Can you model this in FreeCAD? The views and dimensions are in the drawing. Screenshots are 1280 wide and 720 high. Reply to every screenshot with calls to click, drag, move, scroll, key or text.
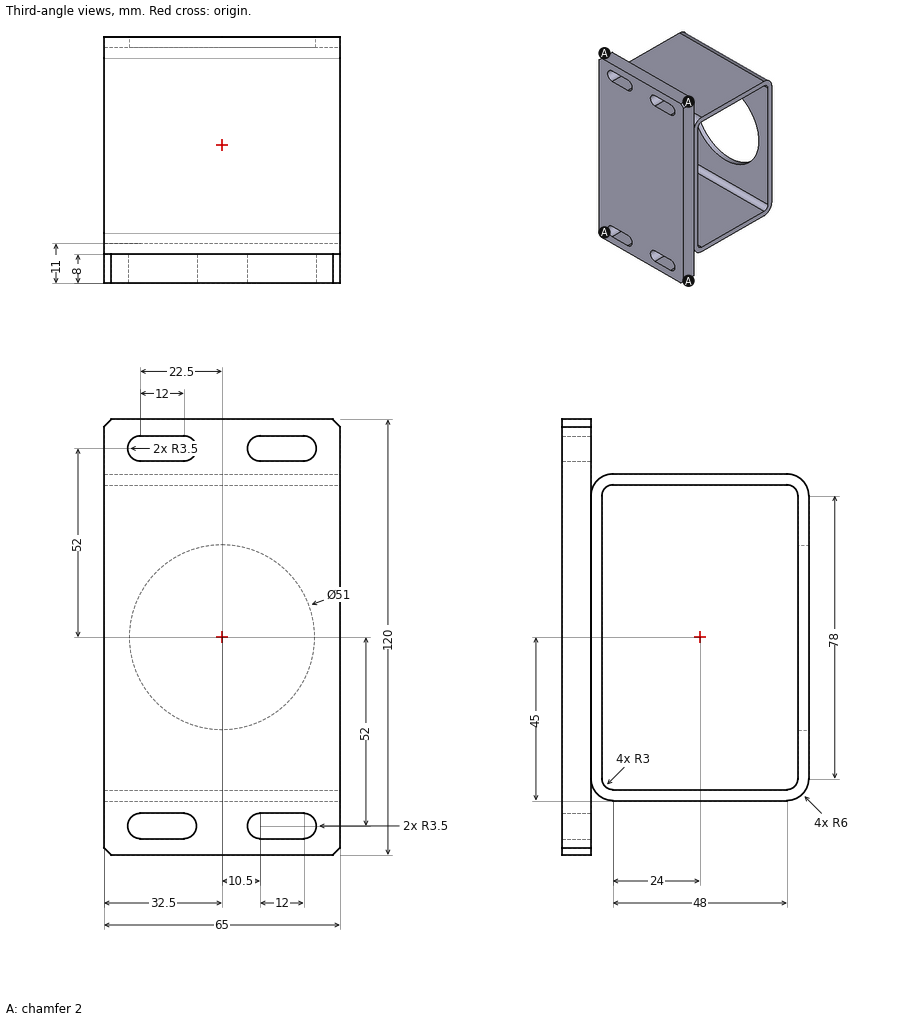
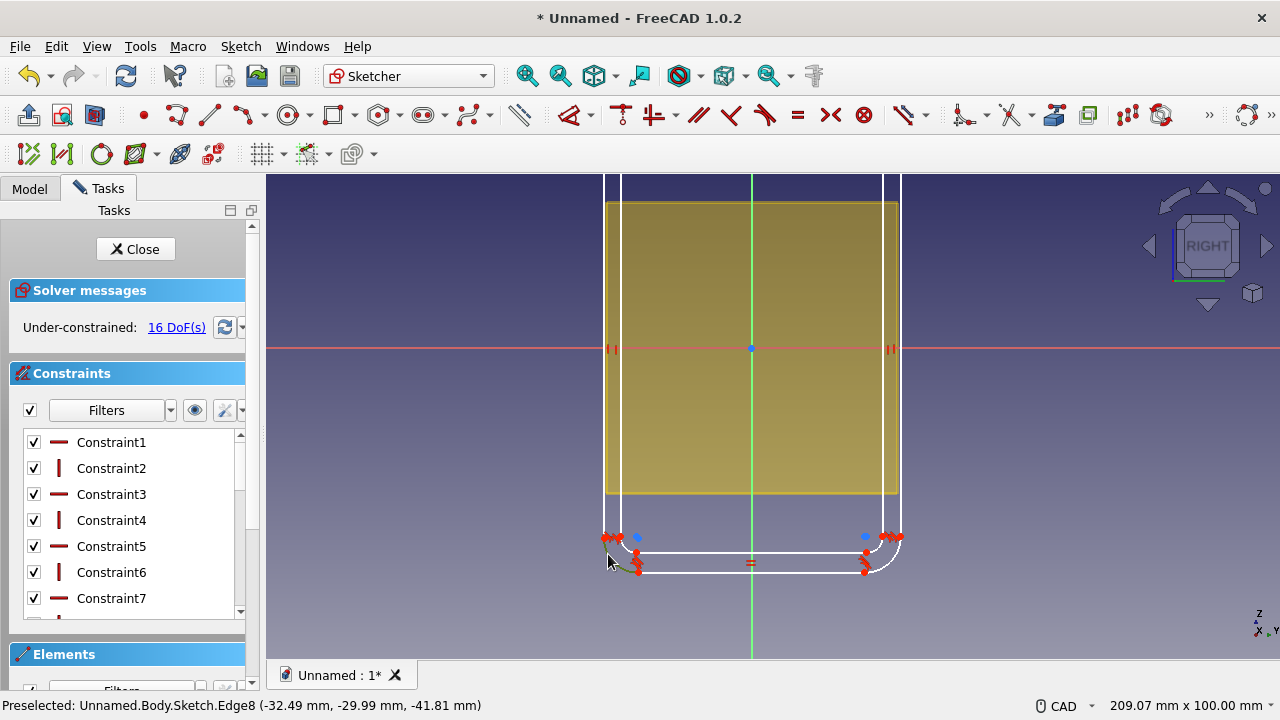
click(625, 548)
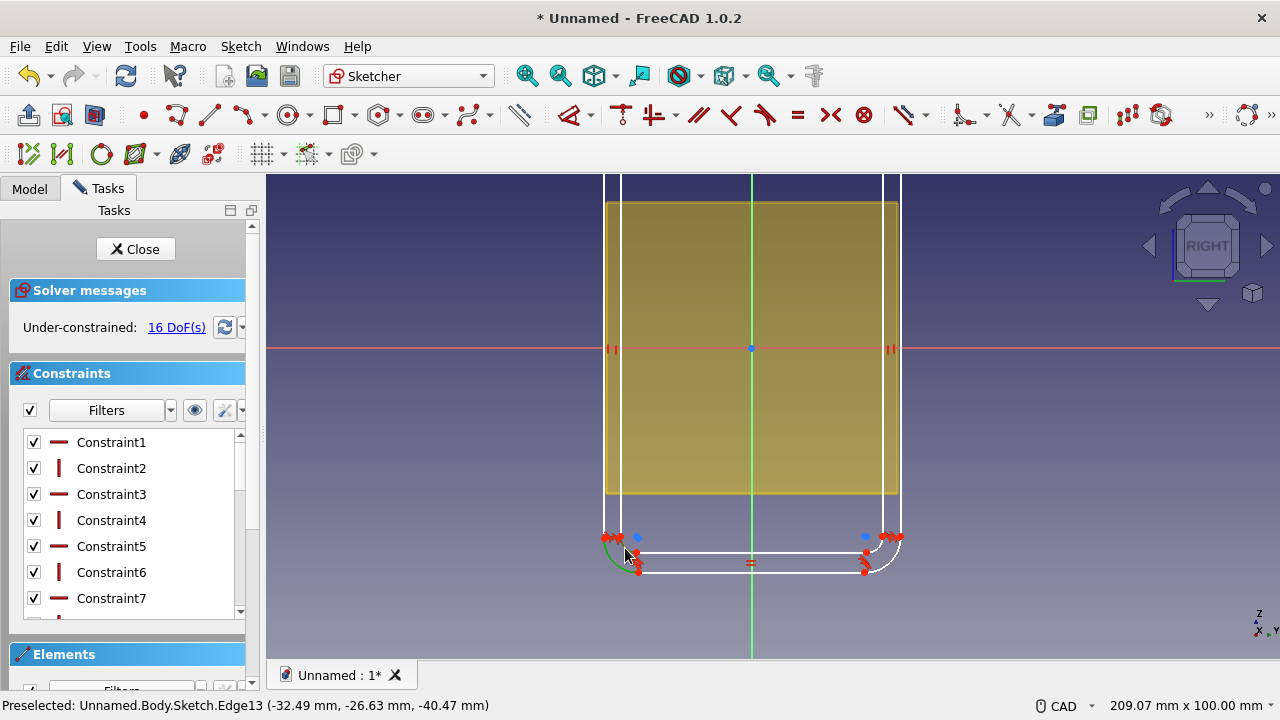
click(621, 116)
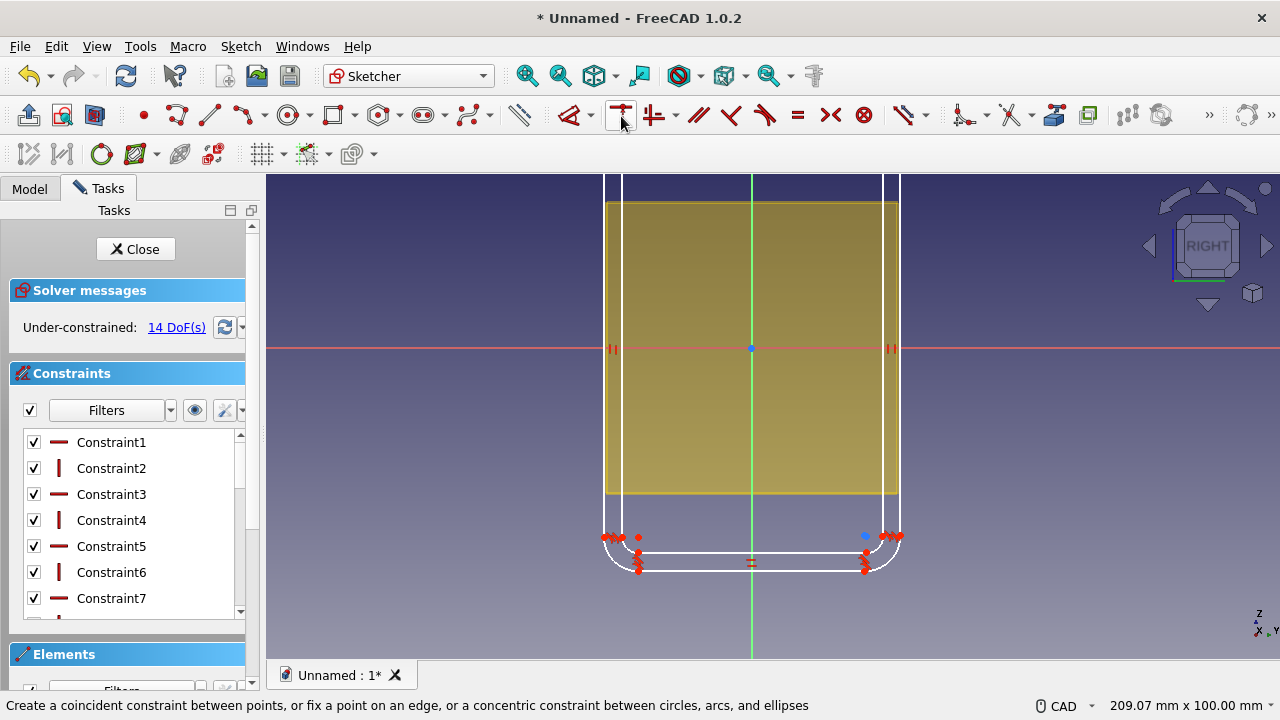
scroll(608, 555, down, 2)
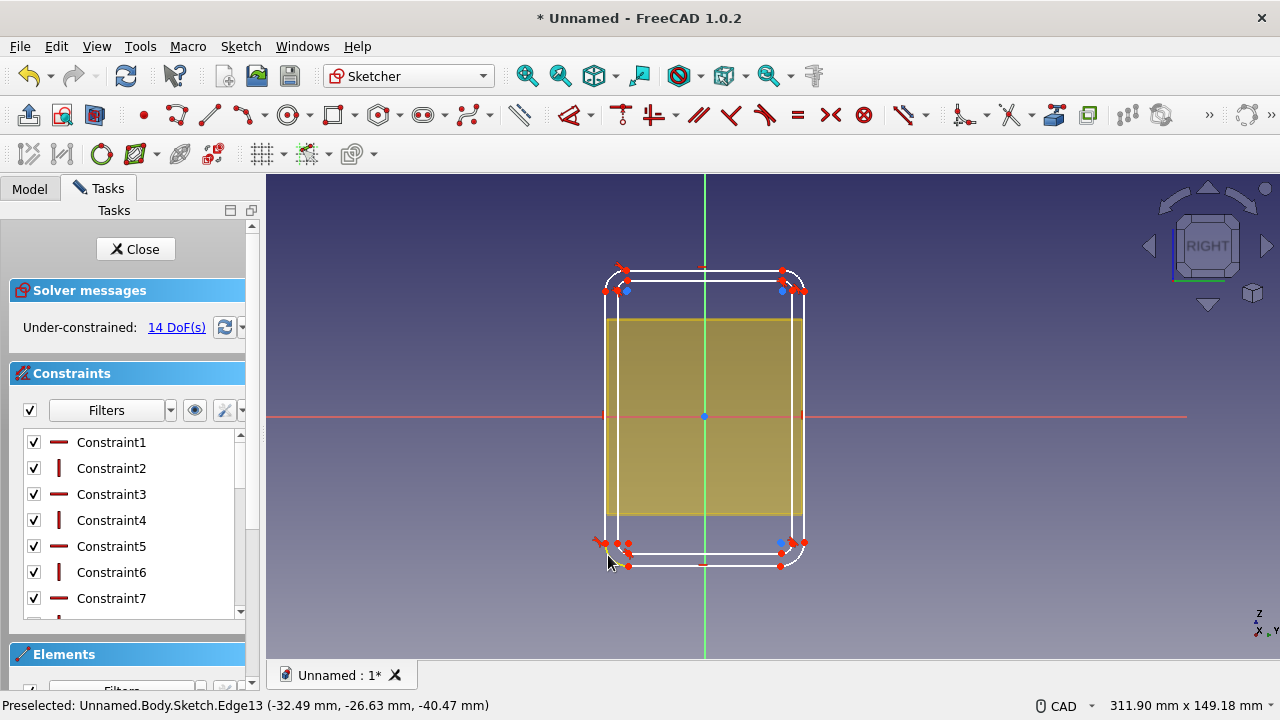
scroll(617, 273, up, 2)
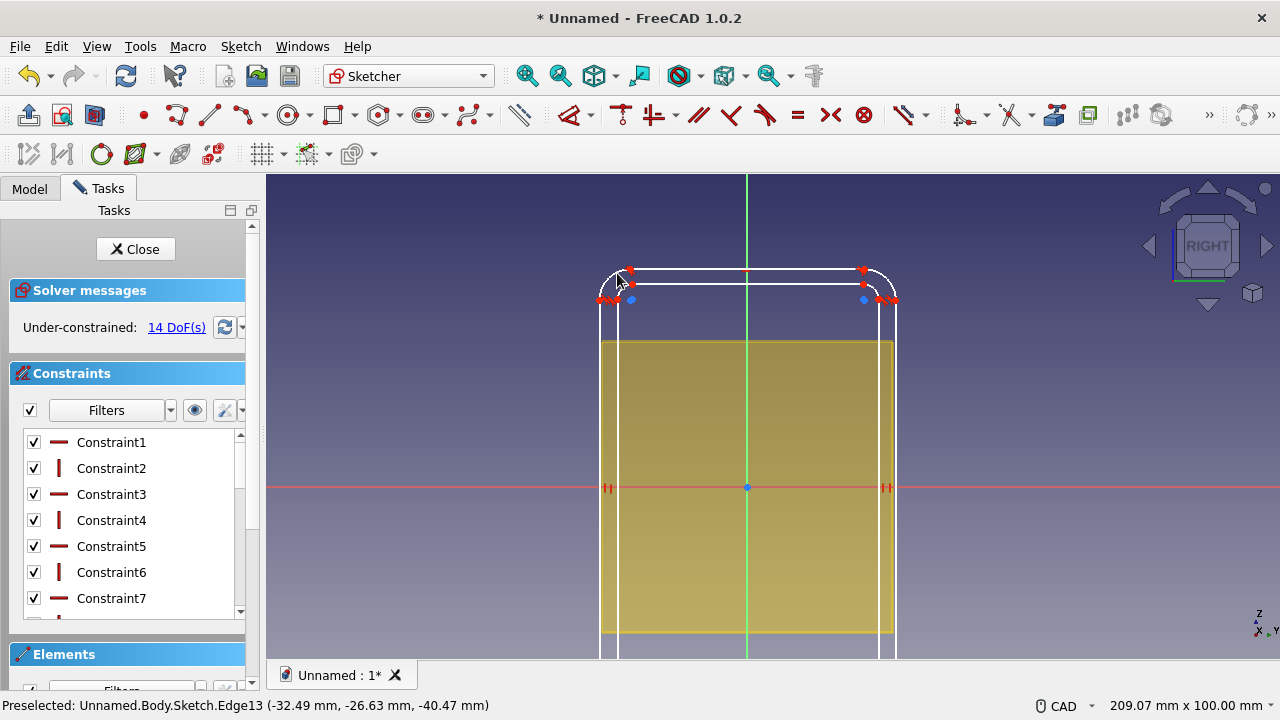
click(616, 273)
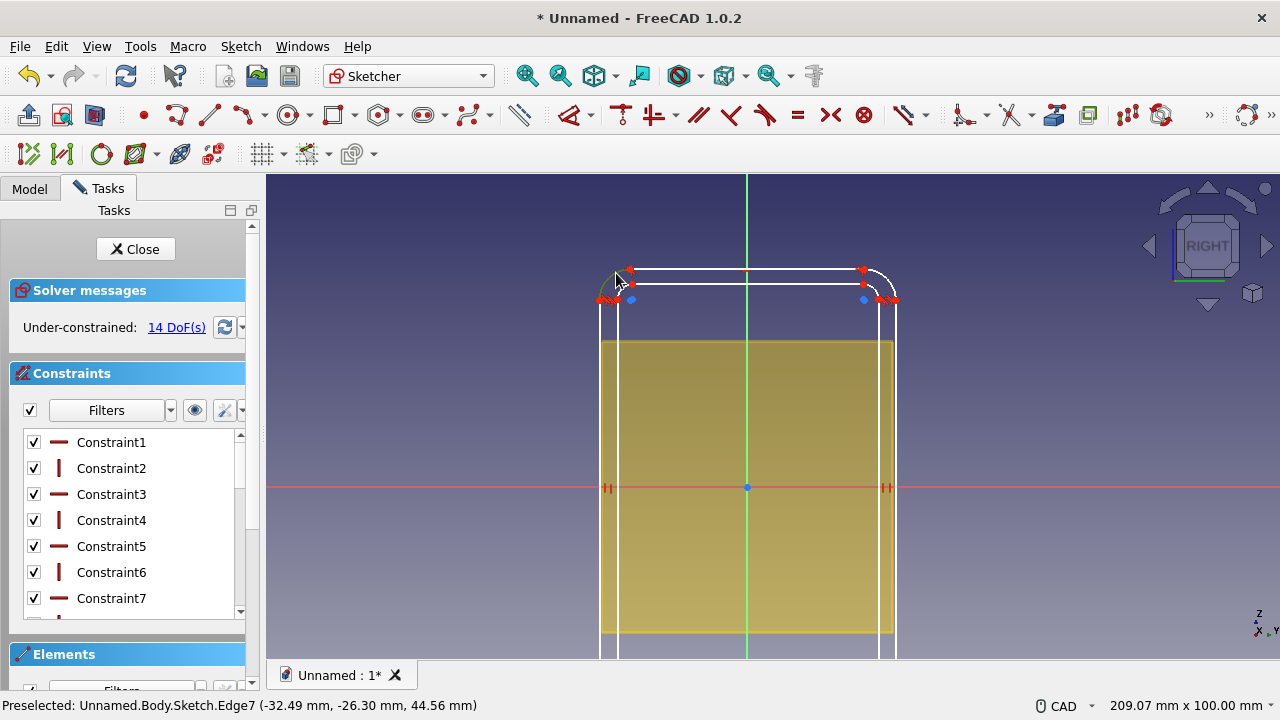
scroll(622, 289, up, 2)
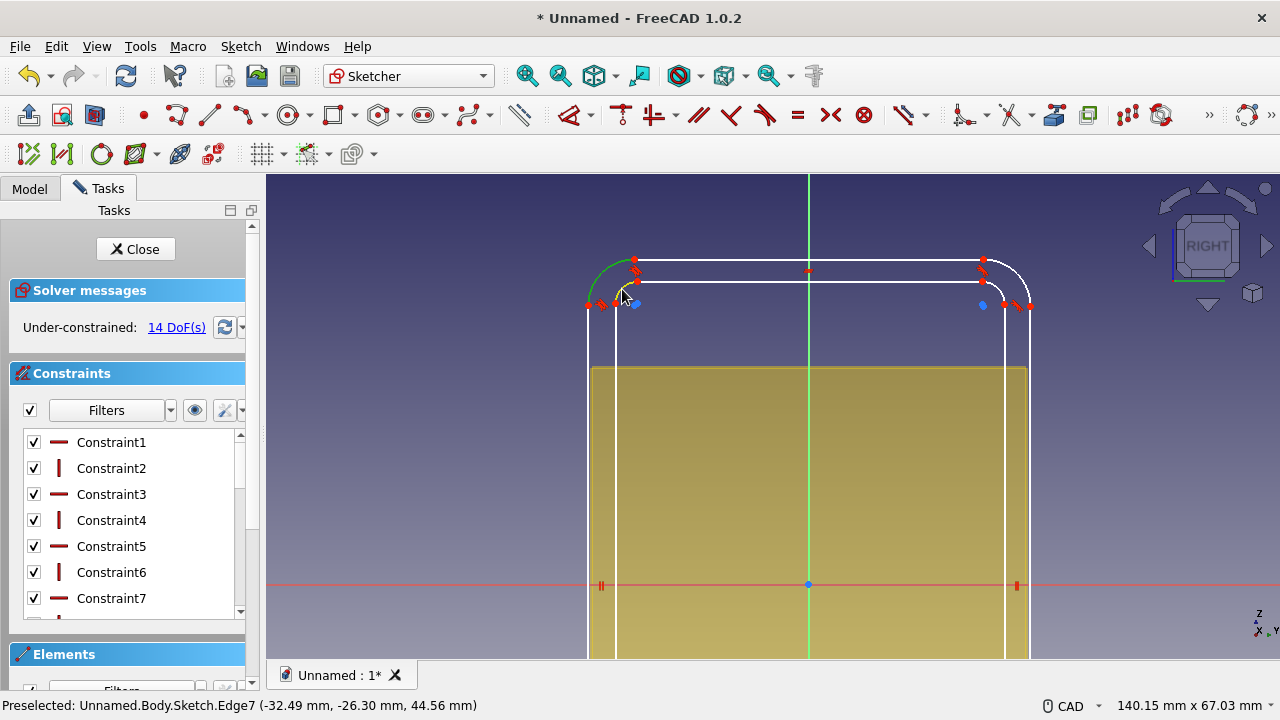
click(622, 288)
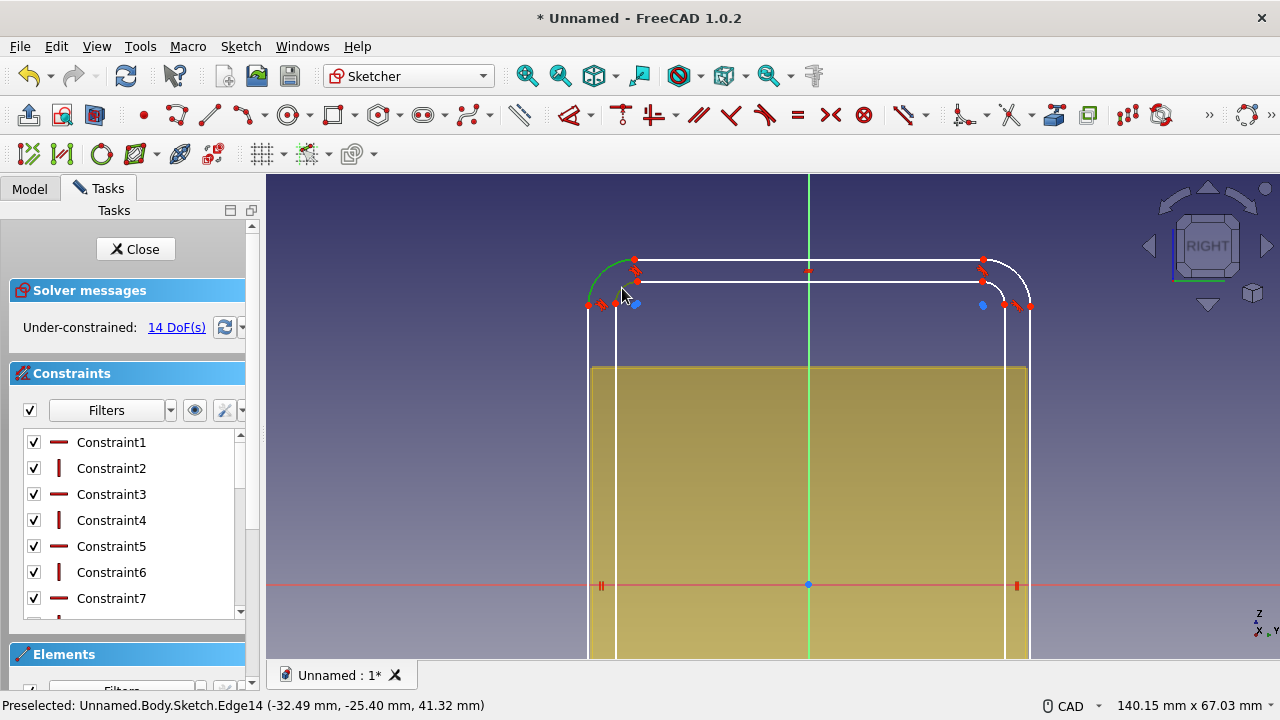
click(621, 116)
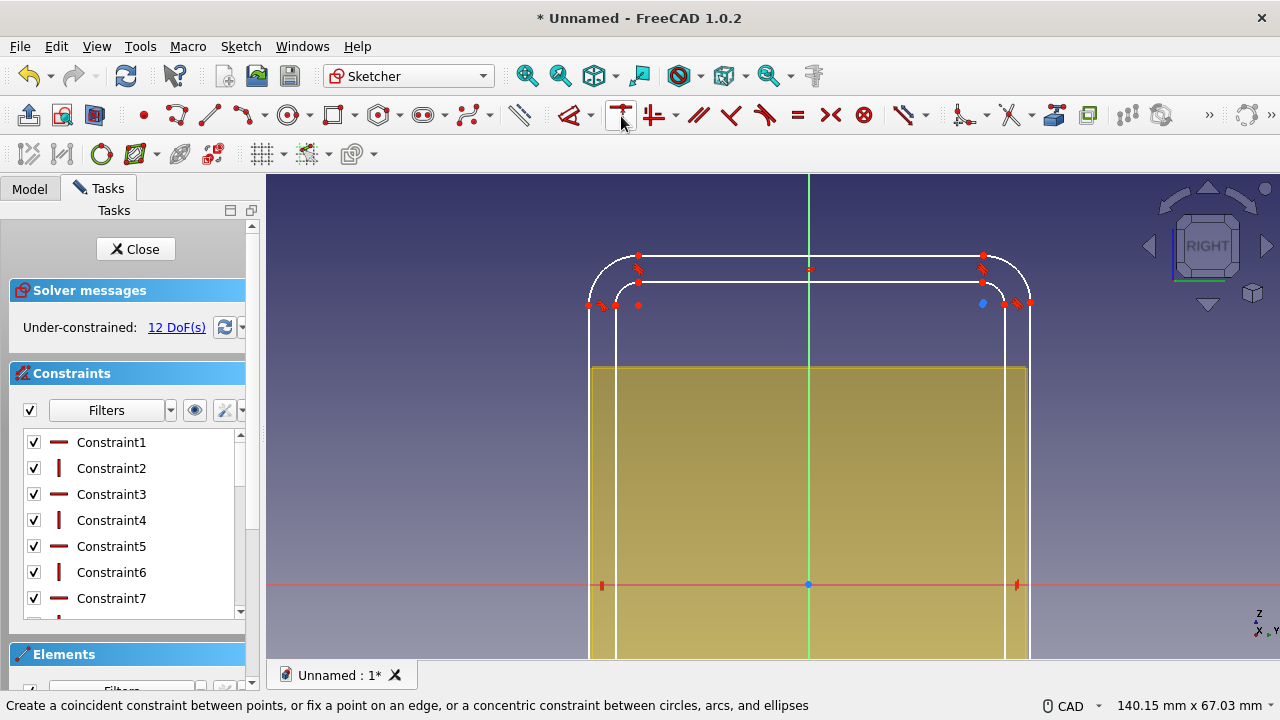
click(1025, 281)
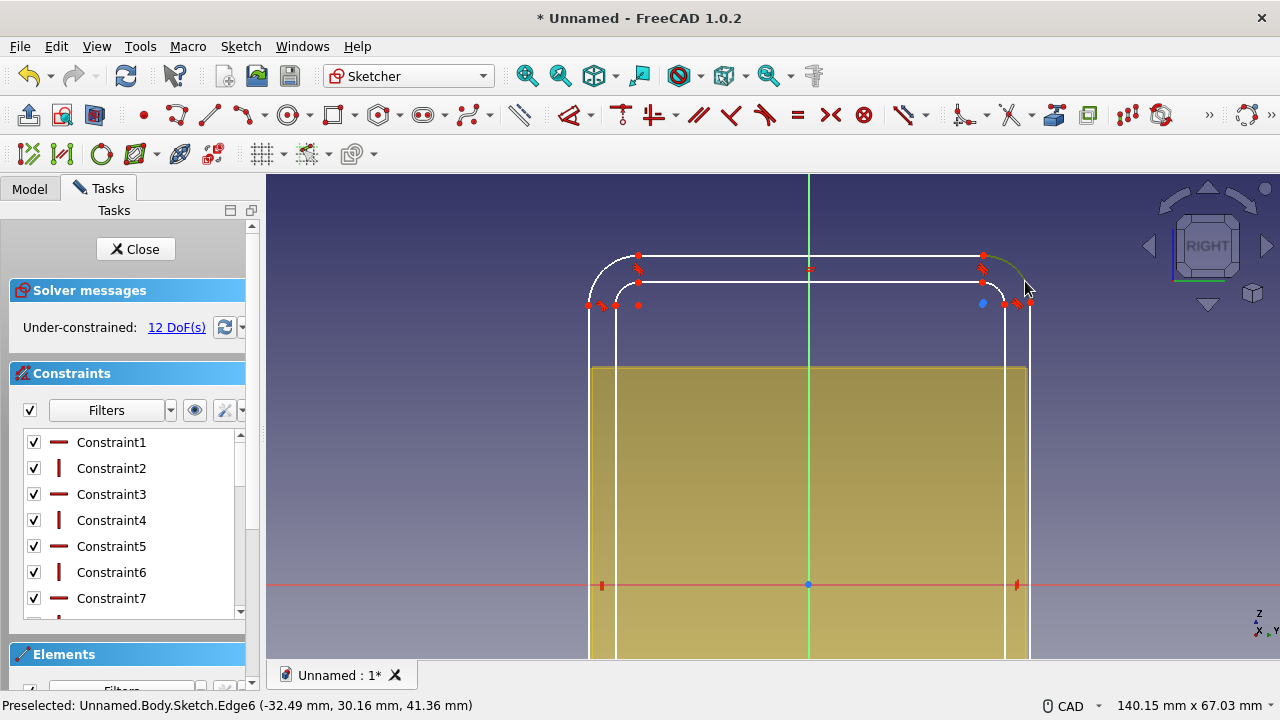
scroll(1002, 295, up, 2)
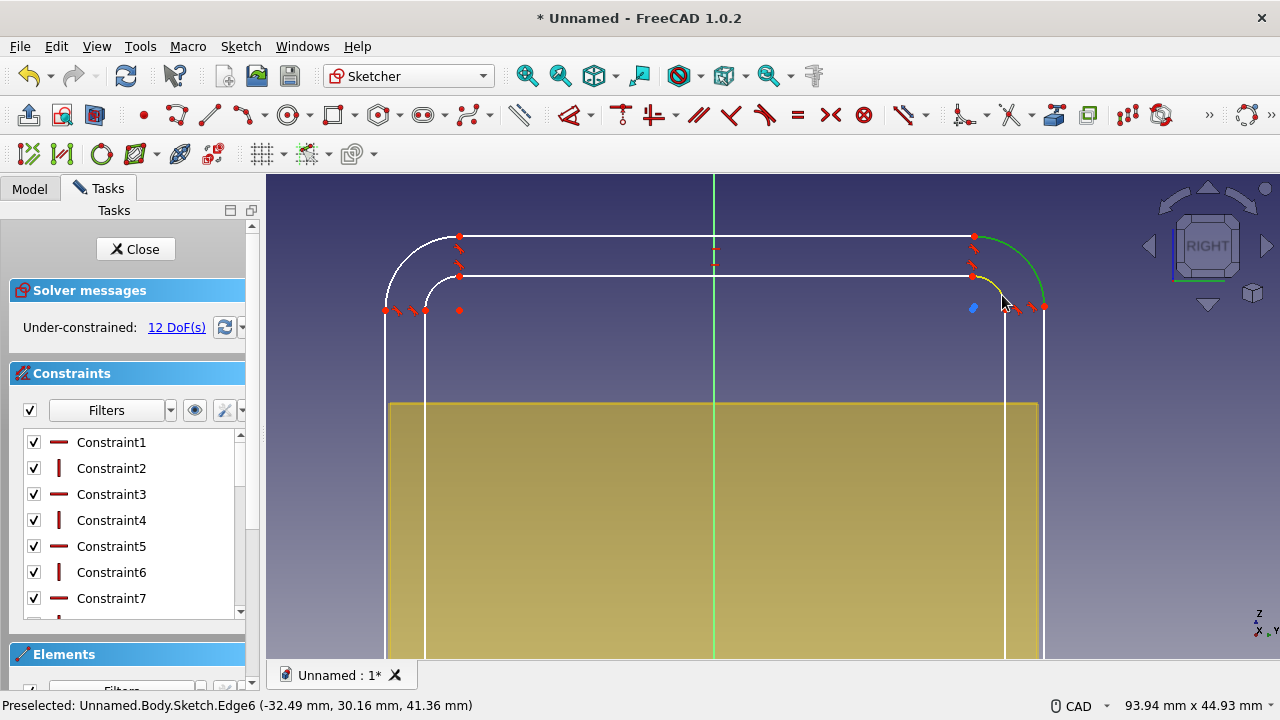
click(1002, 294)